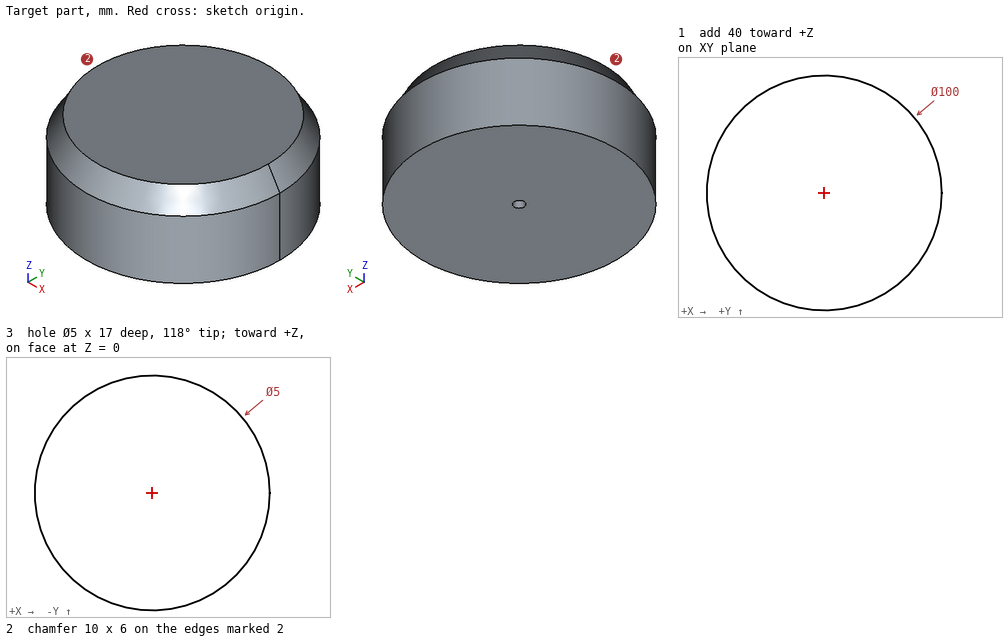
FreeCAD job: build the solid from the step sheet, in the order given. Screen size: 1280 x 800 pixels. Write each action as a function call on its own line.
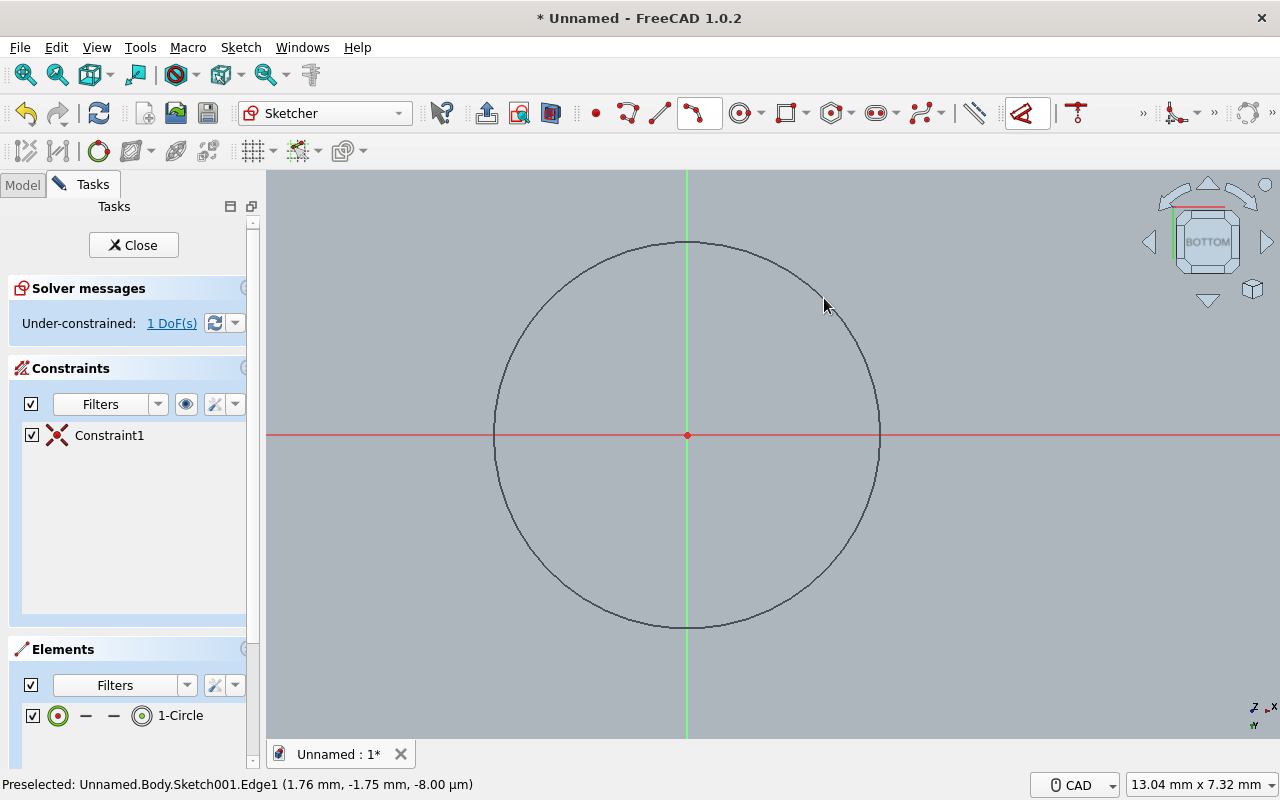
click(823, 298)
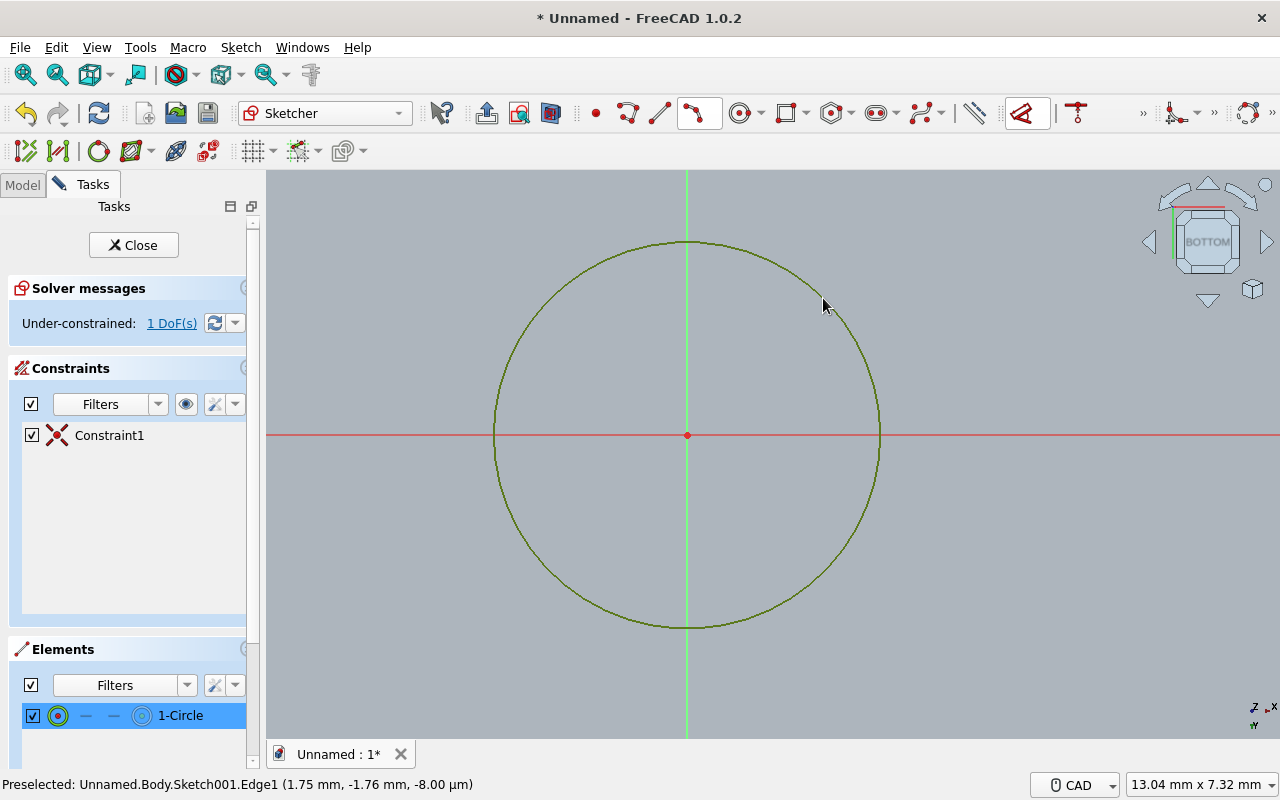
click(1044, 114)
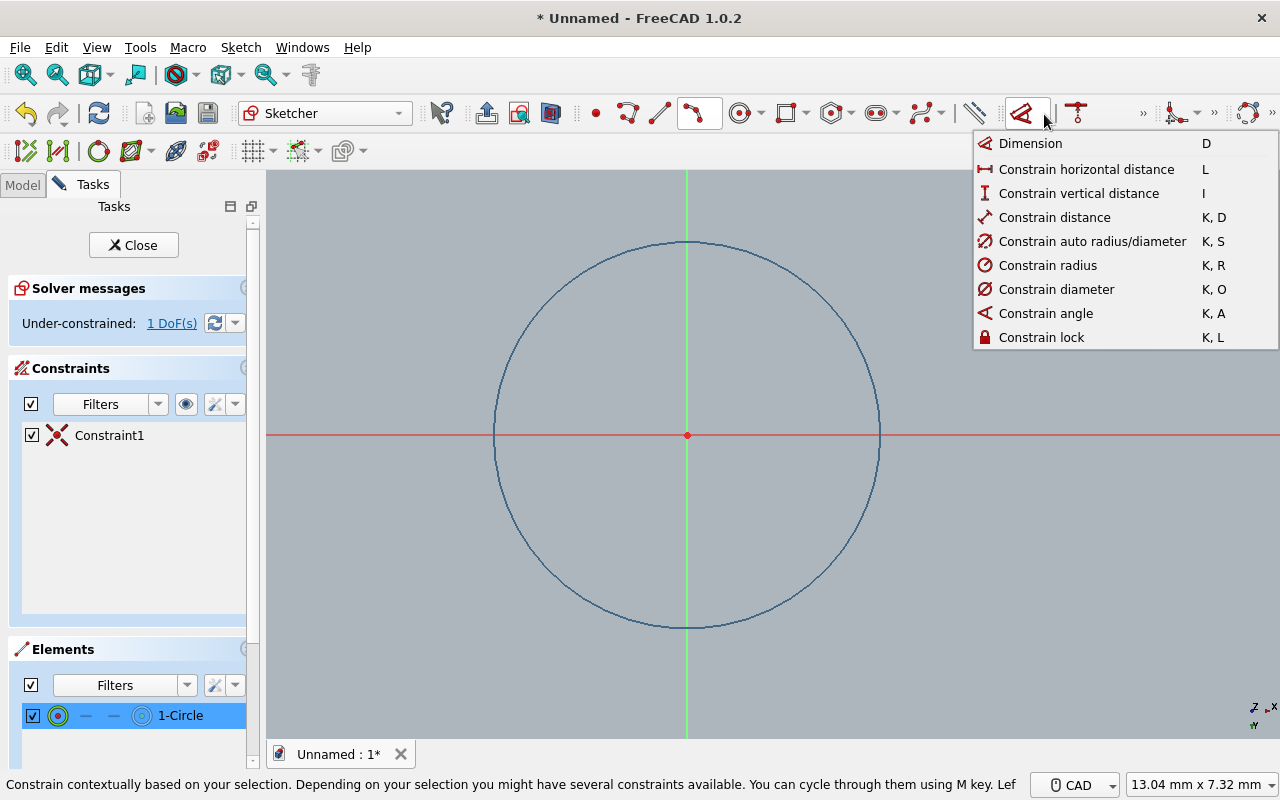
click(1126, 289)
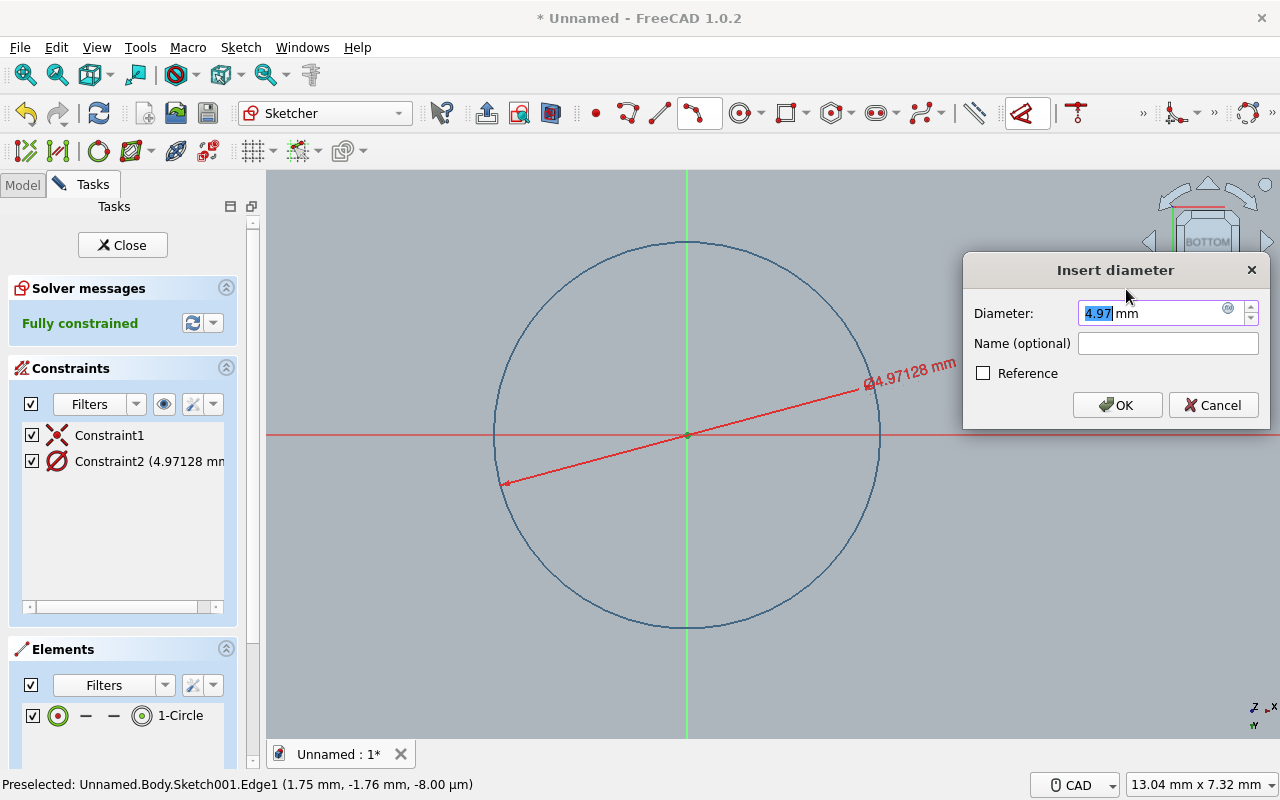
text(5)
key(Return)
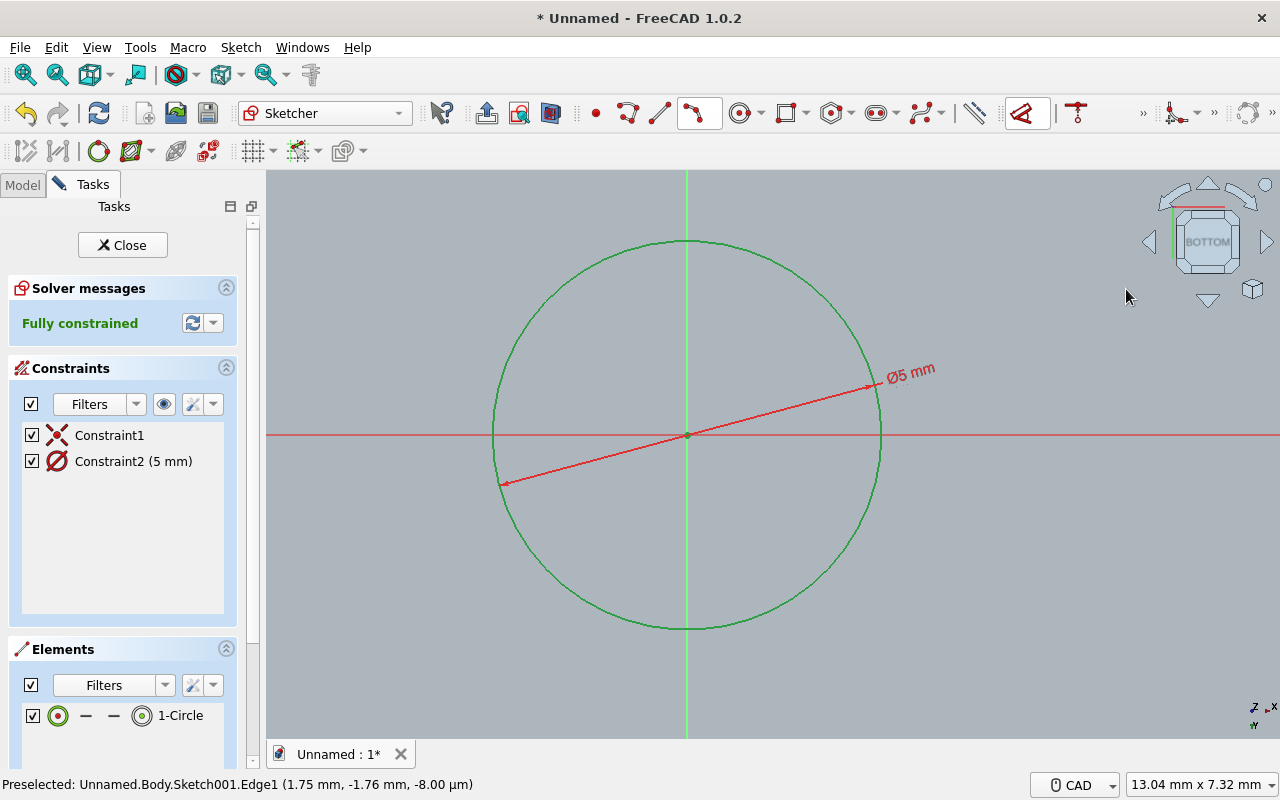
click(123, 245)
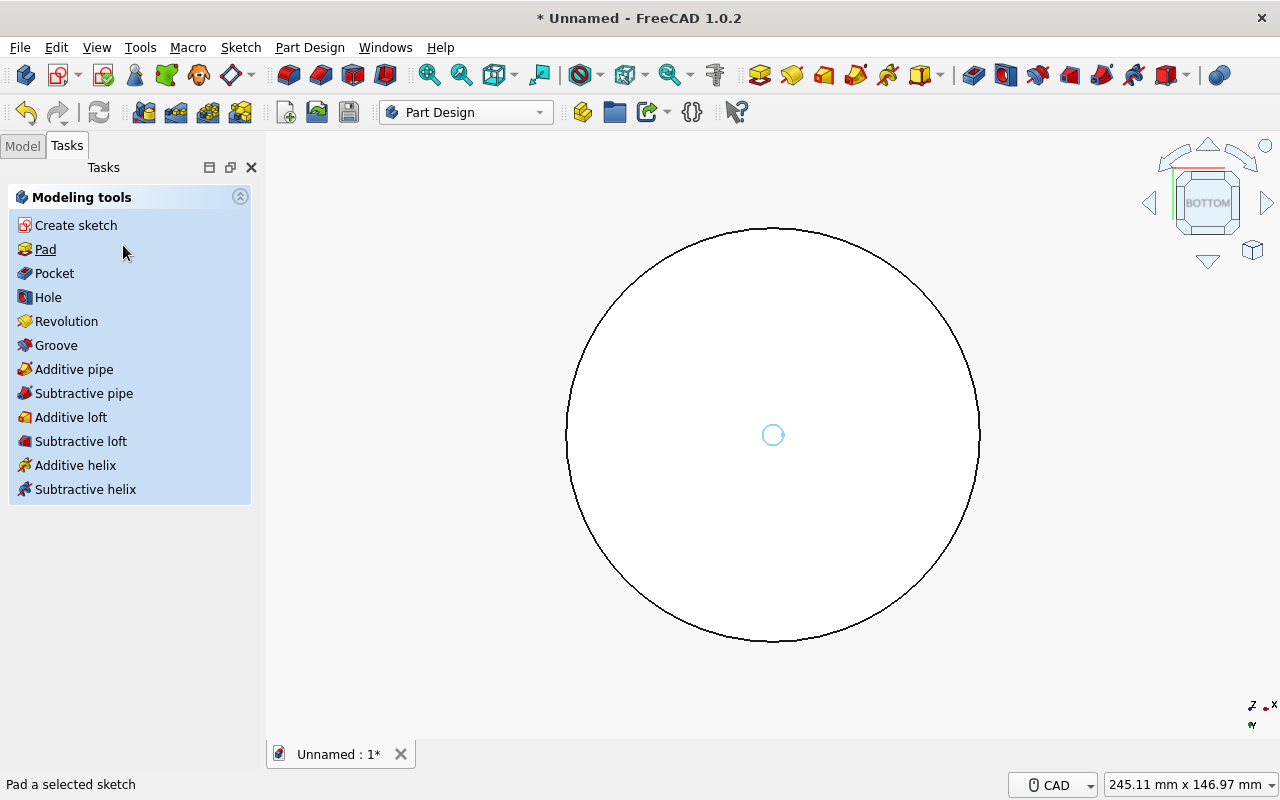
click(1006, 76)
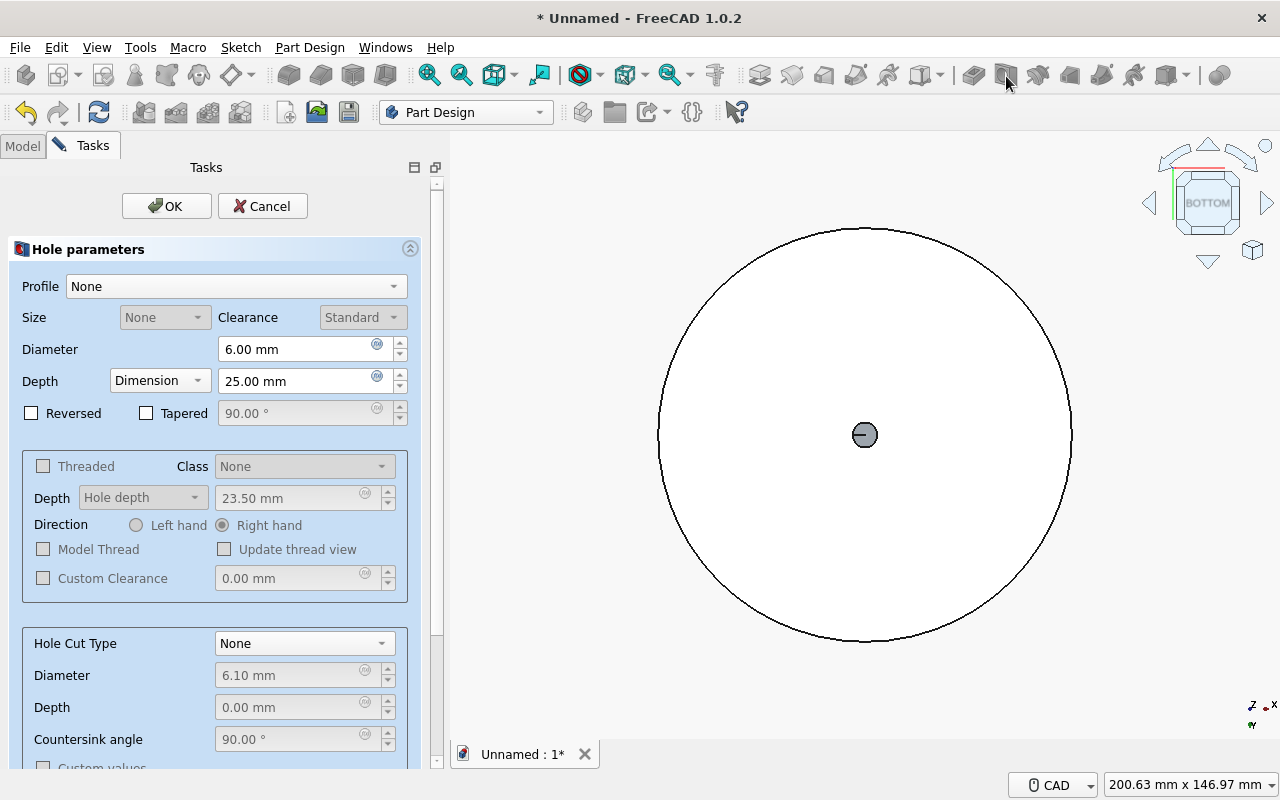
triple_click(305, 349)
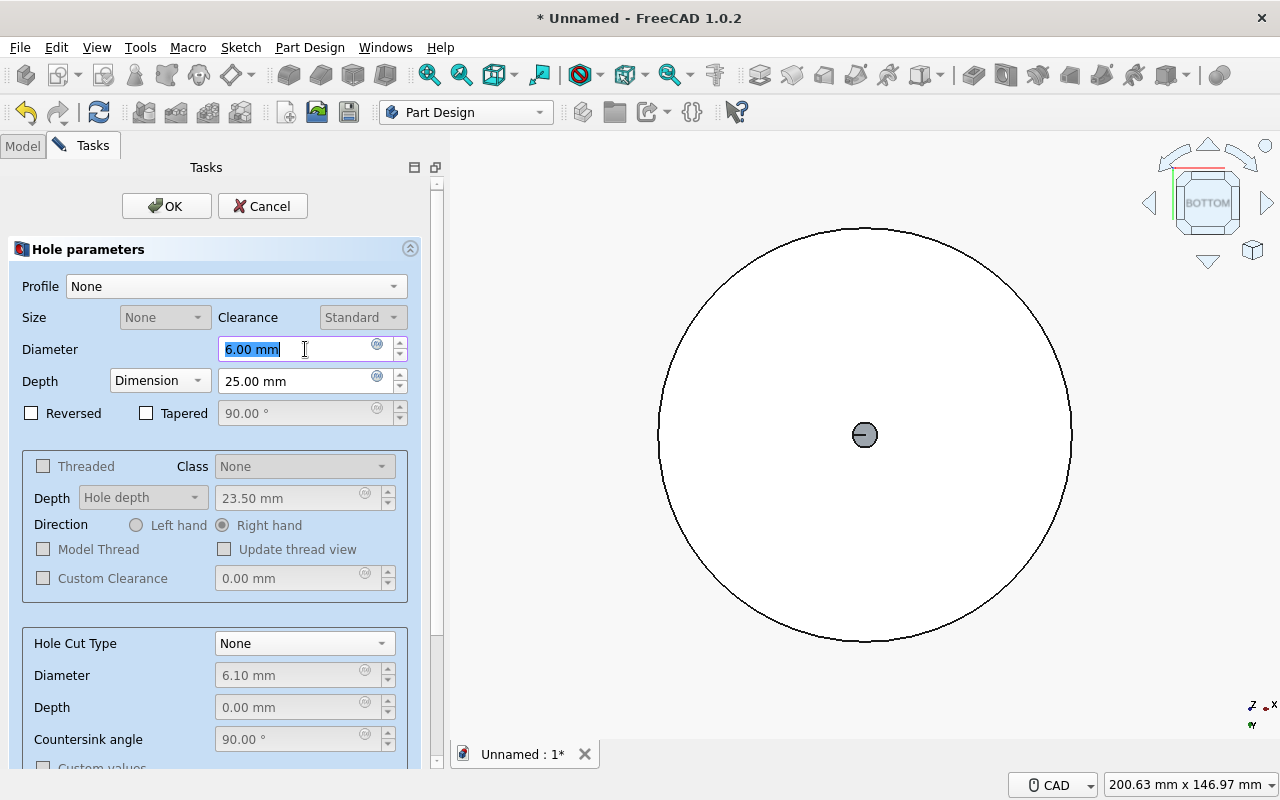
text(5)
key(Tab)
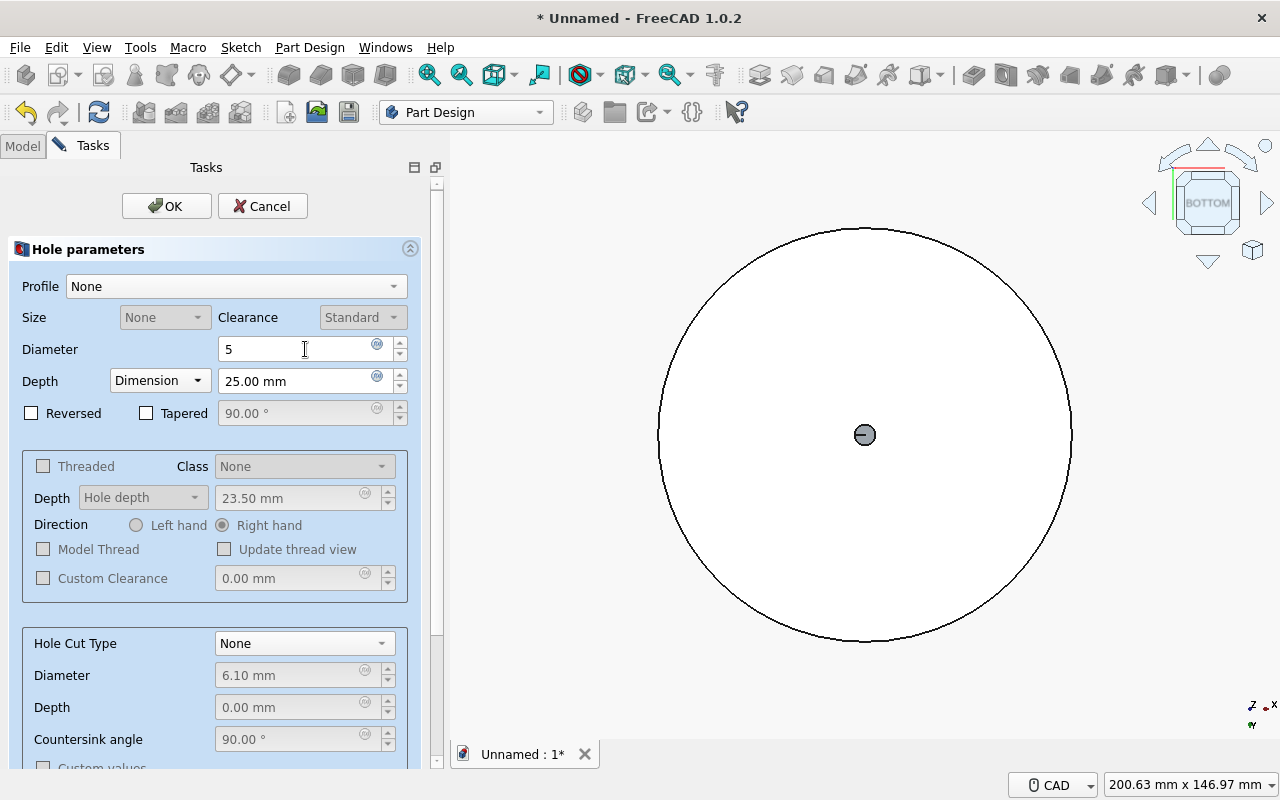
triple_click(305, 381)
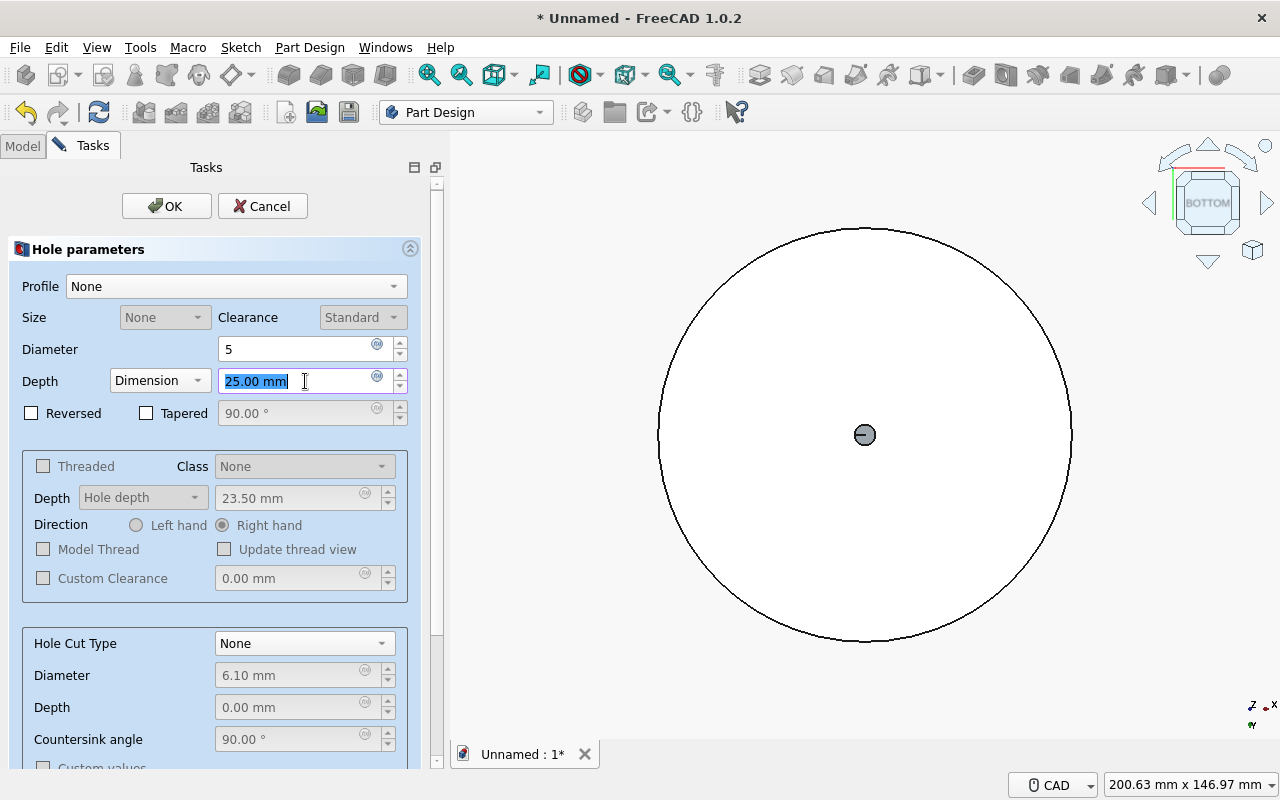
text(17)
key(Tab)